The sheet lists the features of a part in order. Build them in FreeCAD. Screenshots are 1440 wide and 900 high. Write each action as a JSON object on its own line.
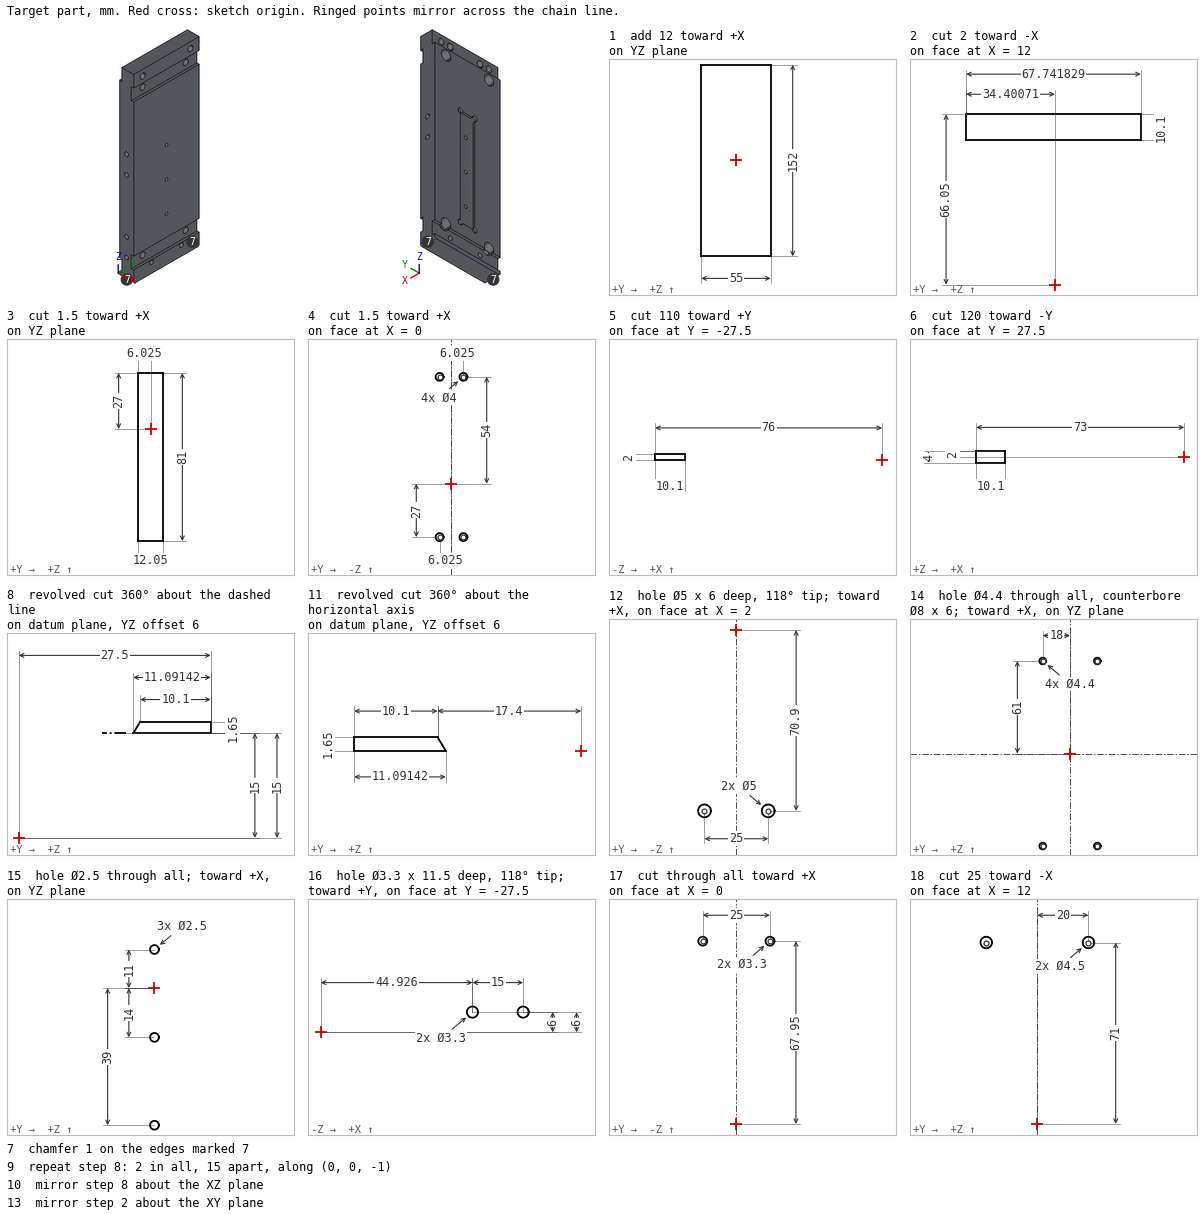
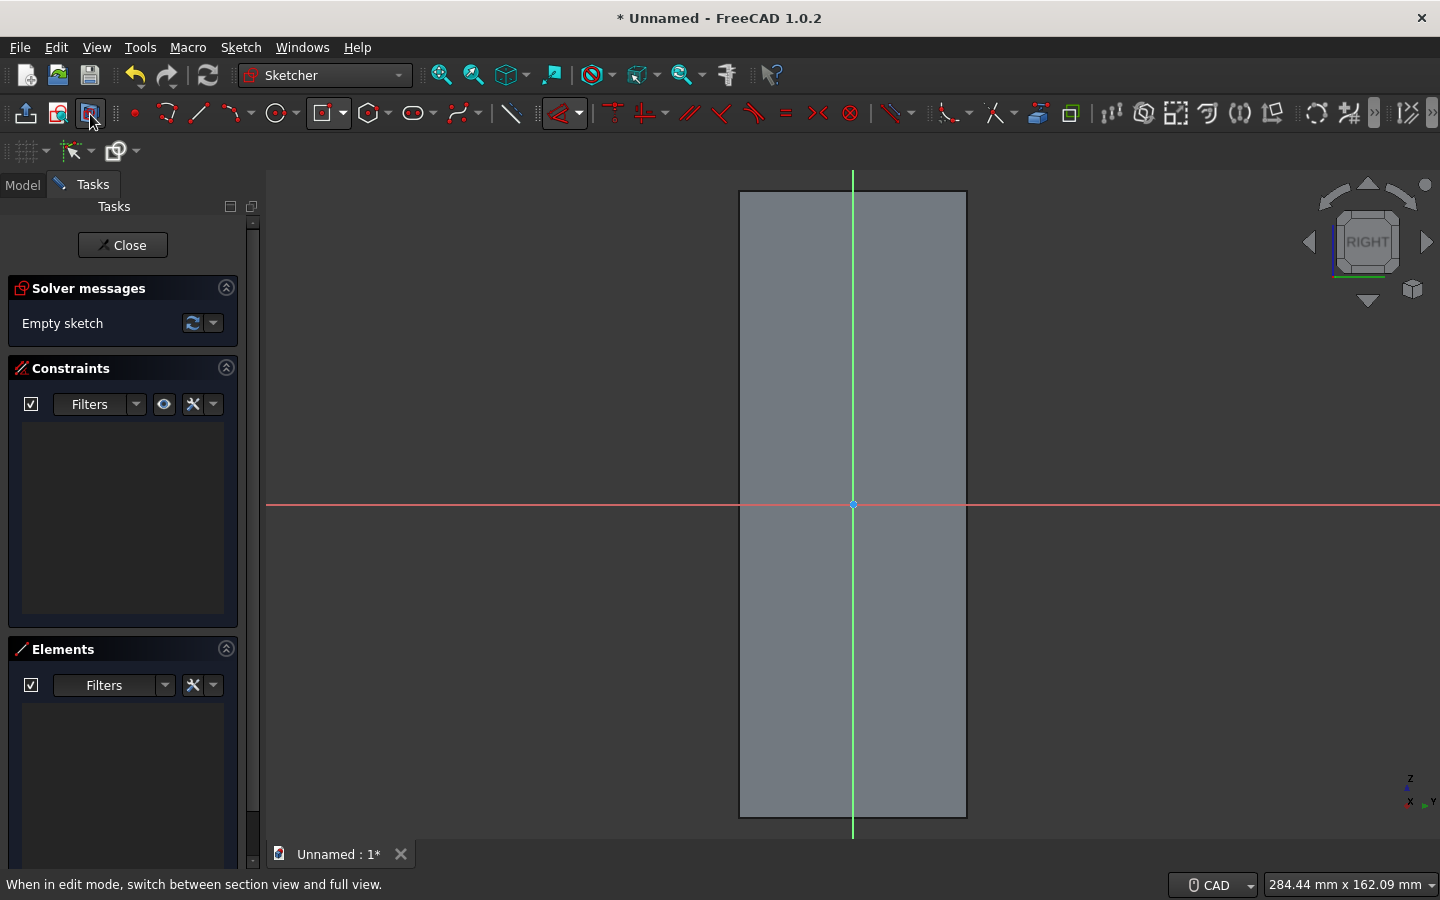
{"action": "key", "text": "g r"}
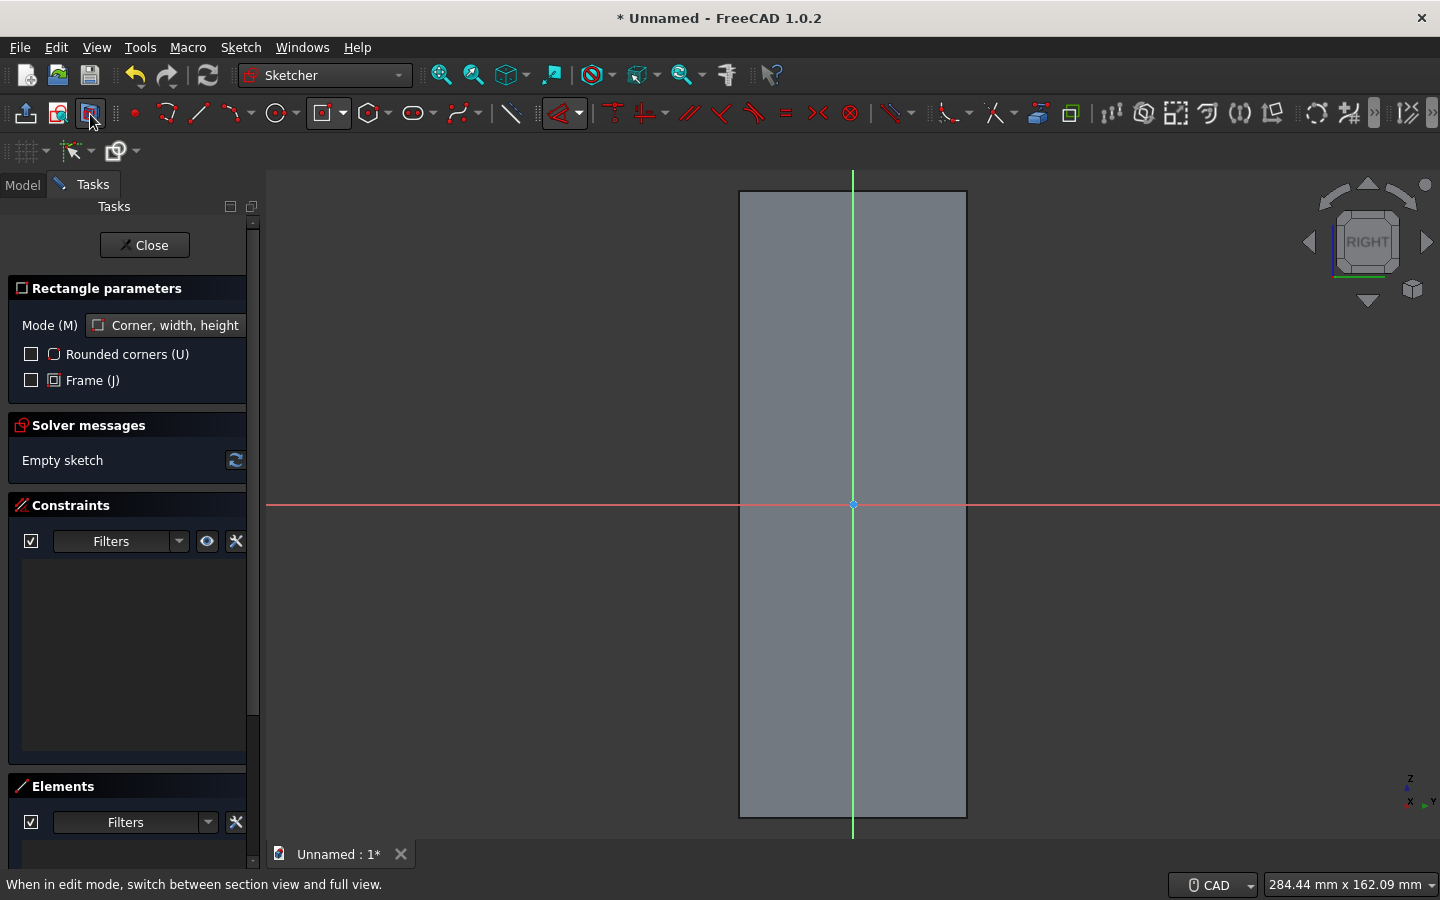
{"action": "left_click", "coordinate": [828, 393]}
{"action": "mouse_move", "coordinate": [878, 727]}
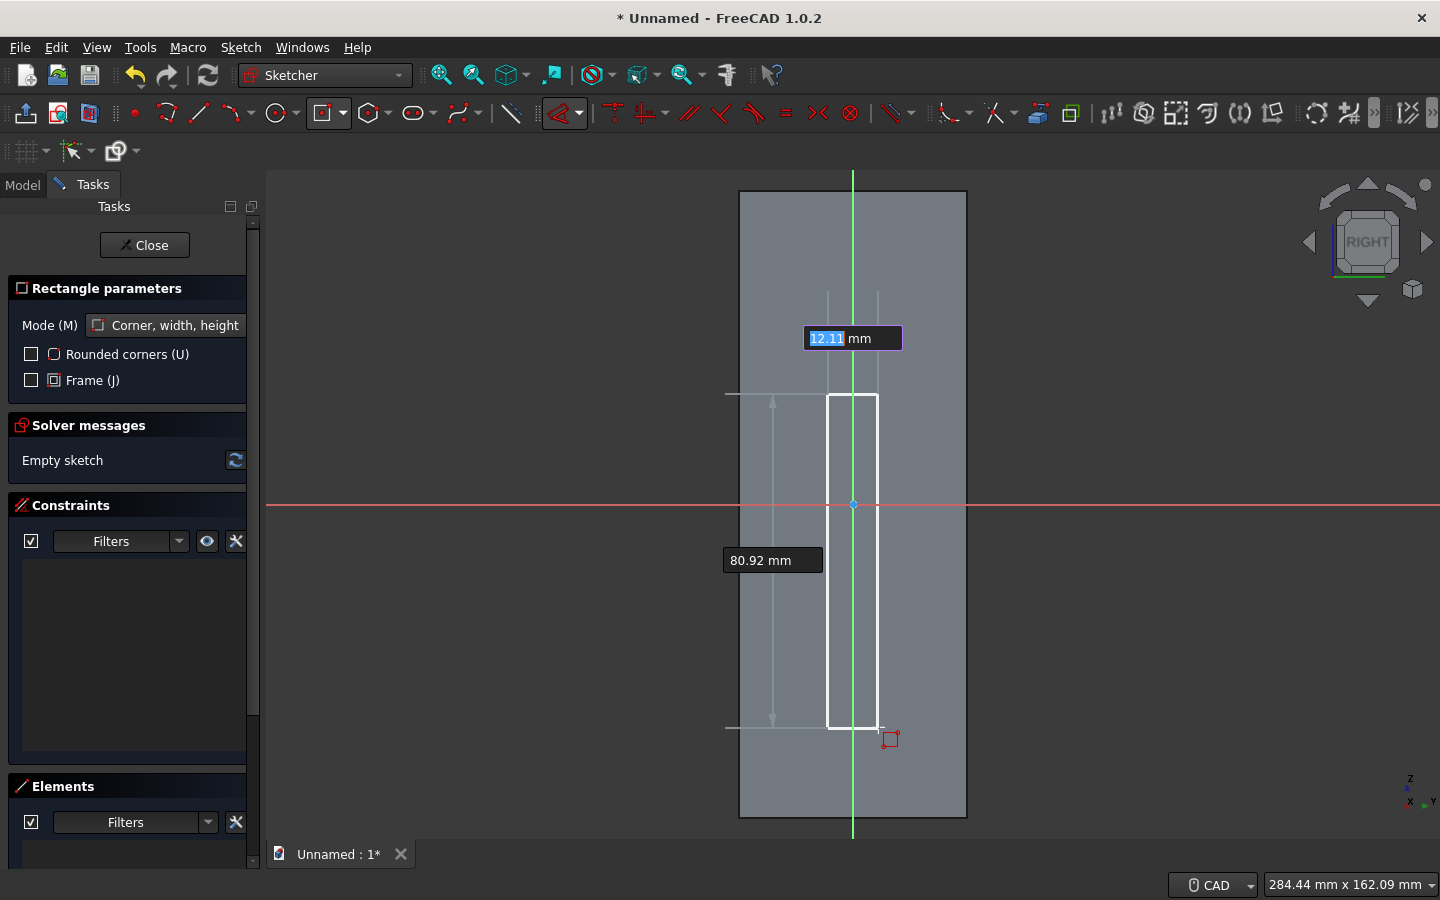
{"action": "type", "text": "12.05"}
{"action": "key", "text": "Tab"}
{"action": "type", "text": "81"}
{"action": "key", "text": "Return"}
{"action": "key", "text": "Escape"}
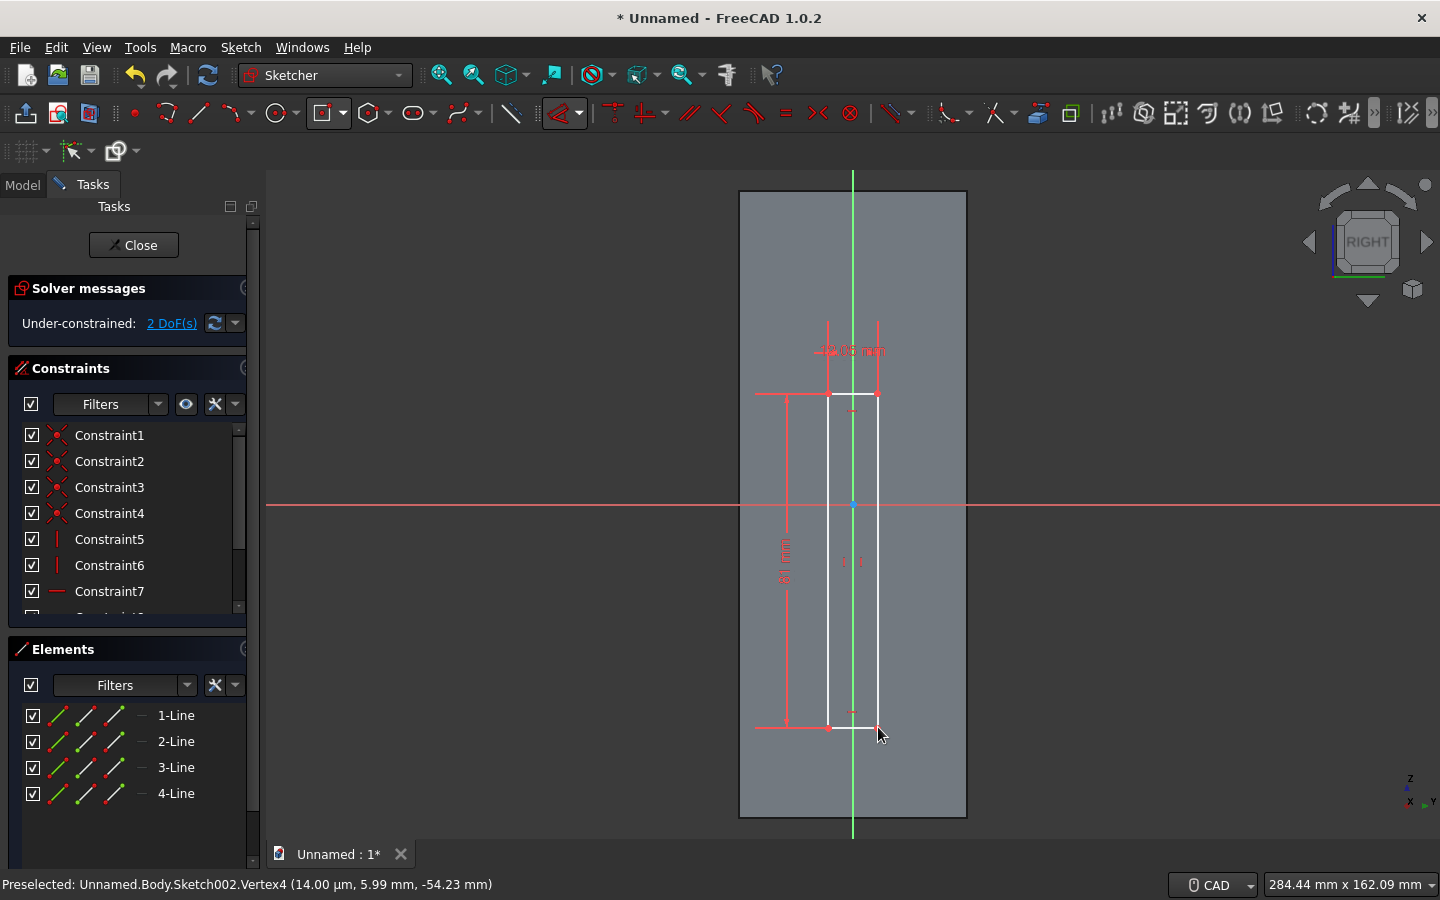
{"action": "left_click", "coordinate": [828, 394]}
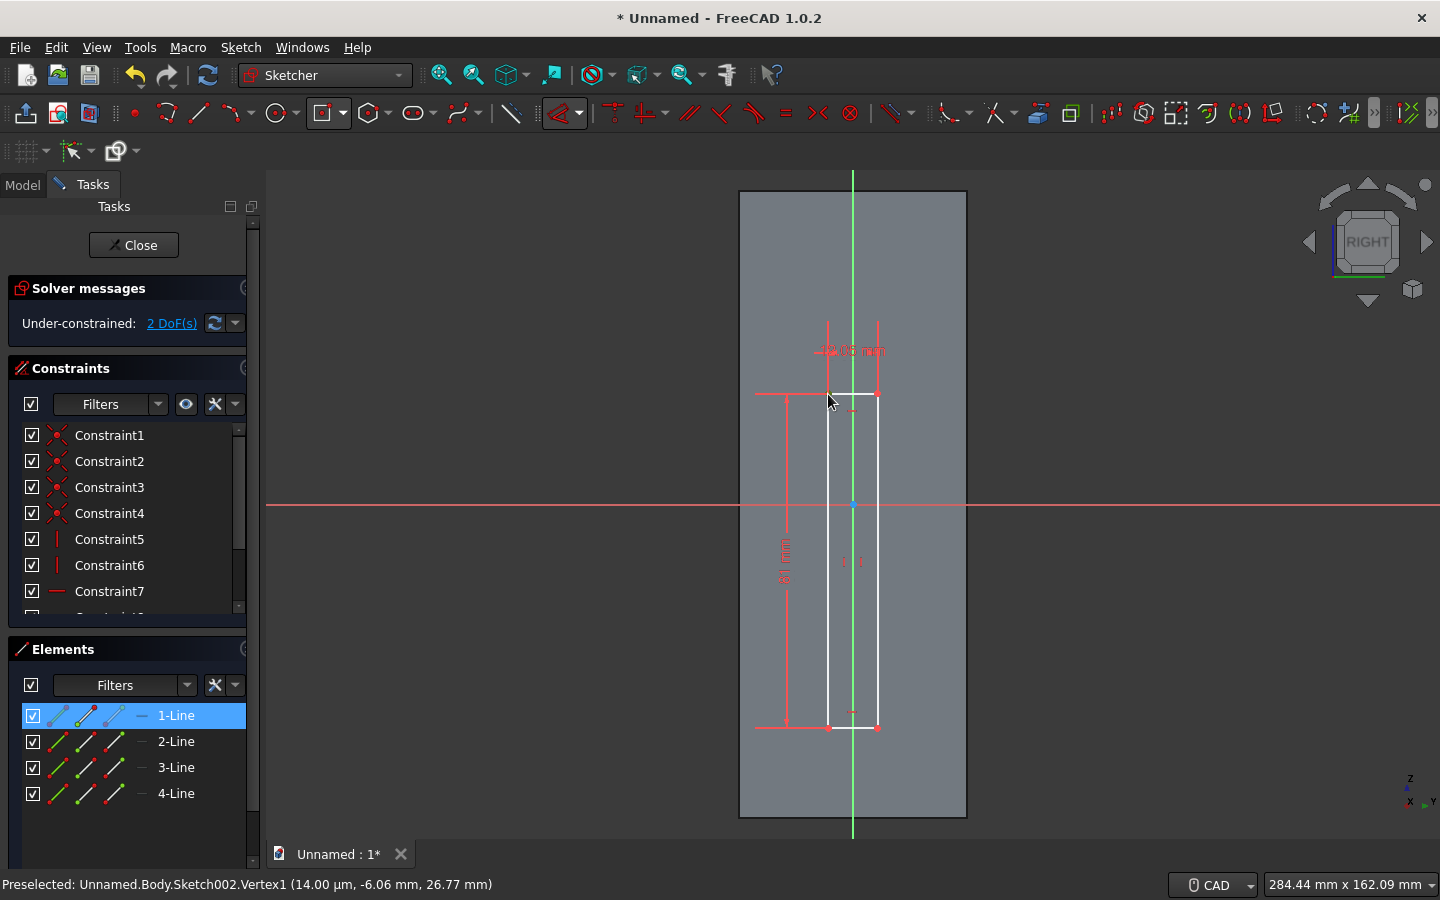
{"action": "left_click", "coordinate": [582, 114]}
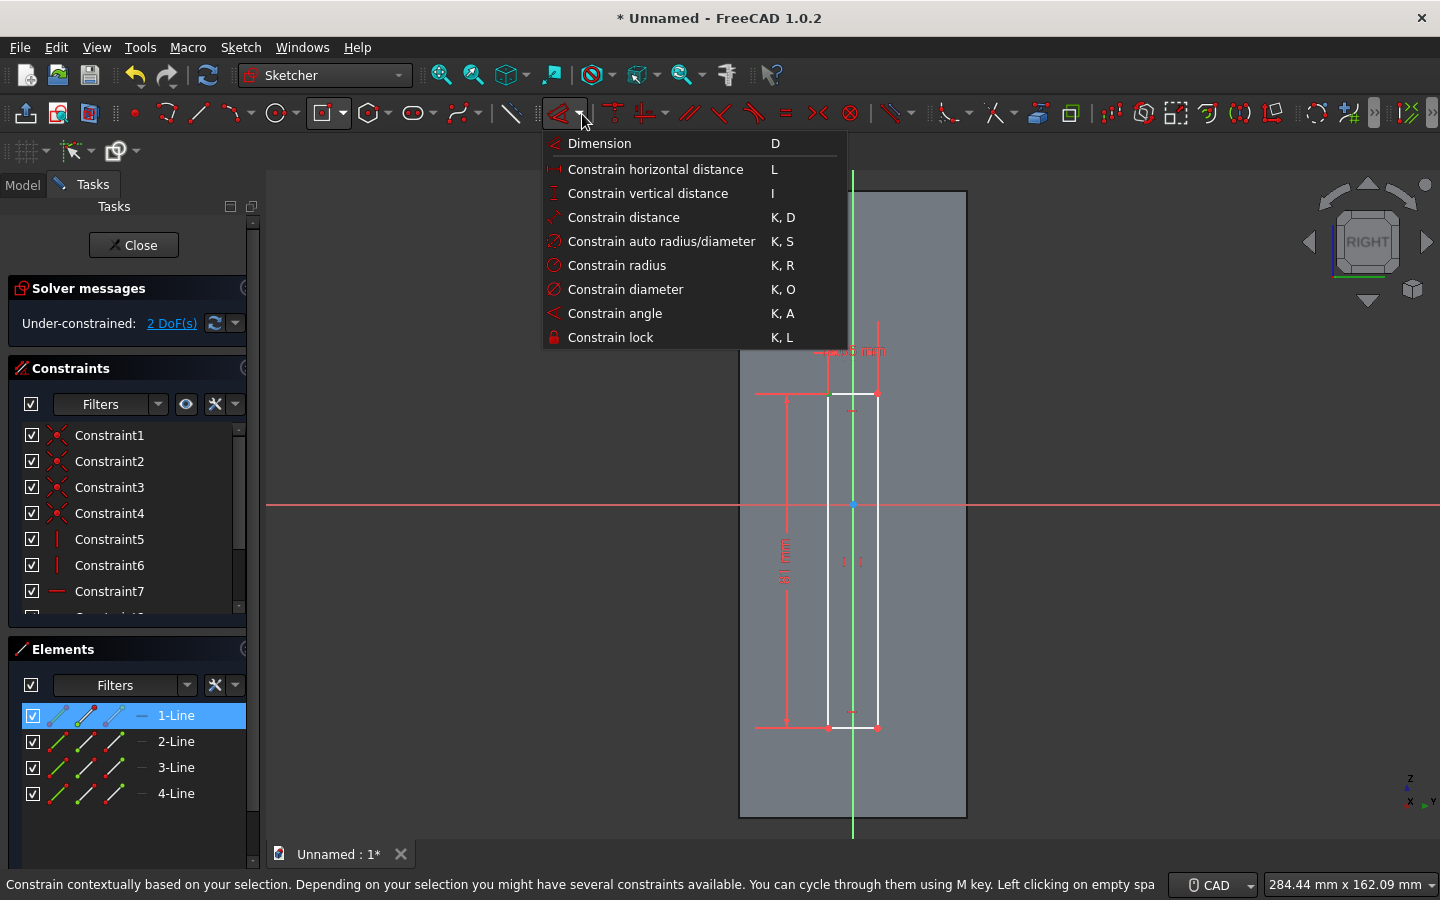
{"action": "left_click", "coordinate": [695, 193]}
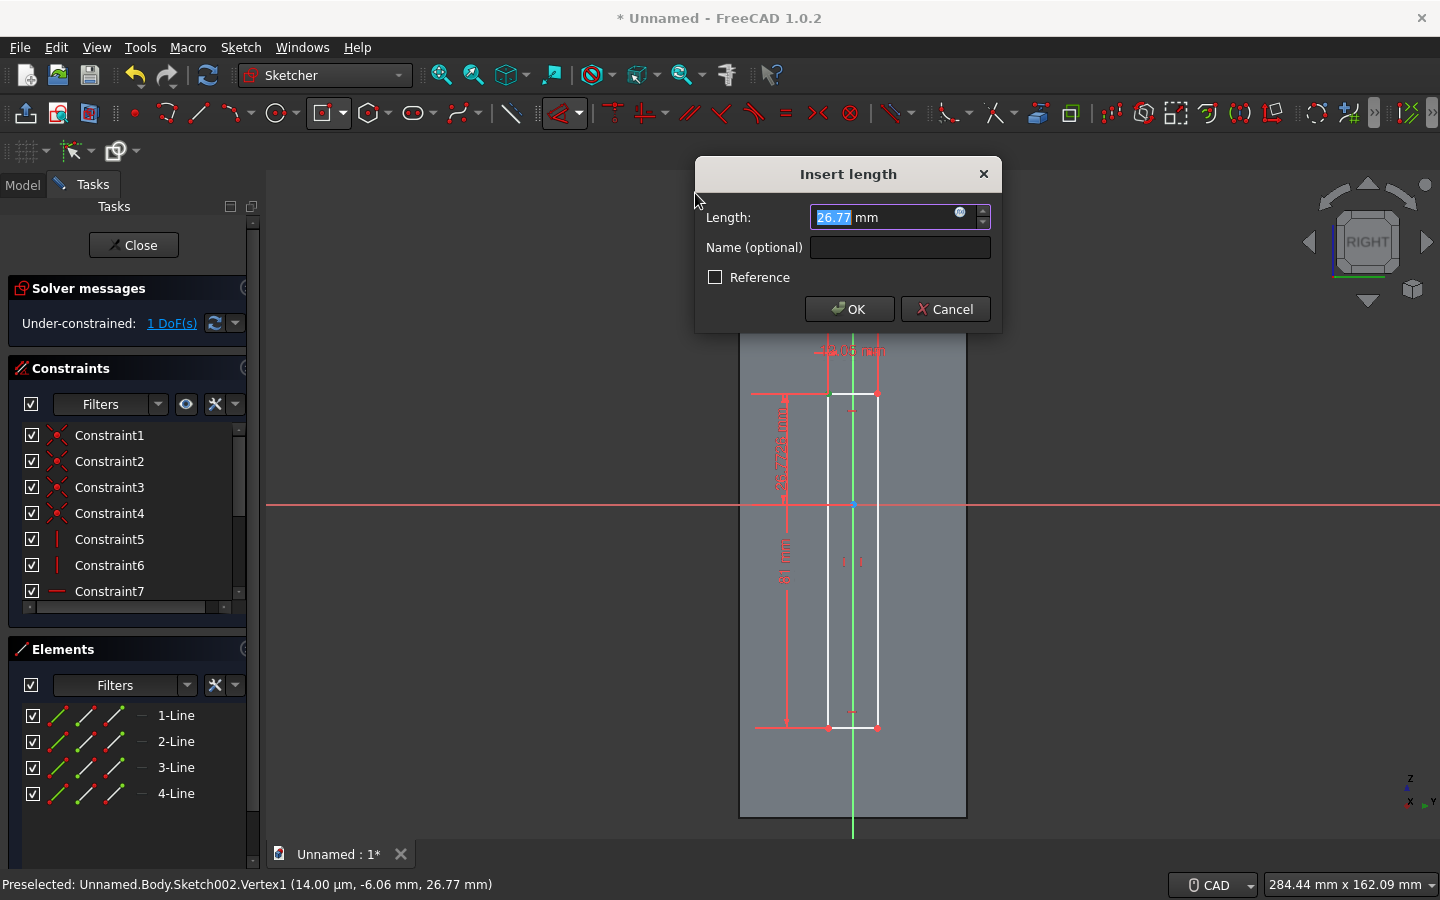
{"action": "type", "text": "27"}
{"action": "key", "text": "Return"}